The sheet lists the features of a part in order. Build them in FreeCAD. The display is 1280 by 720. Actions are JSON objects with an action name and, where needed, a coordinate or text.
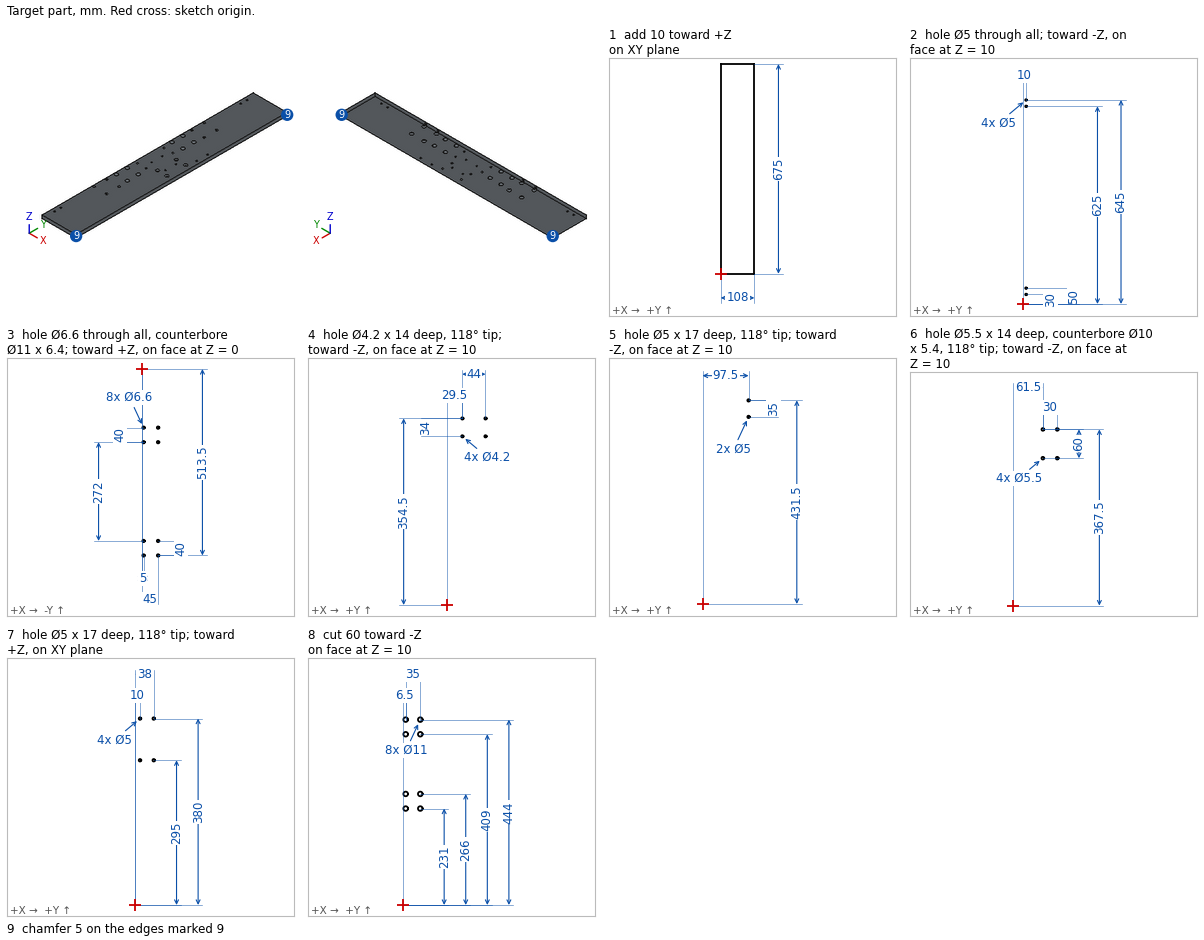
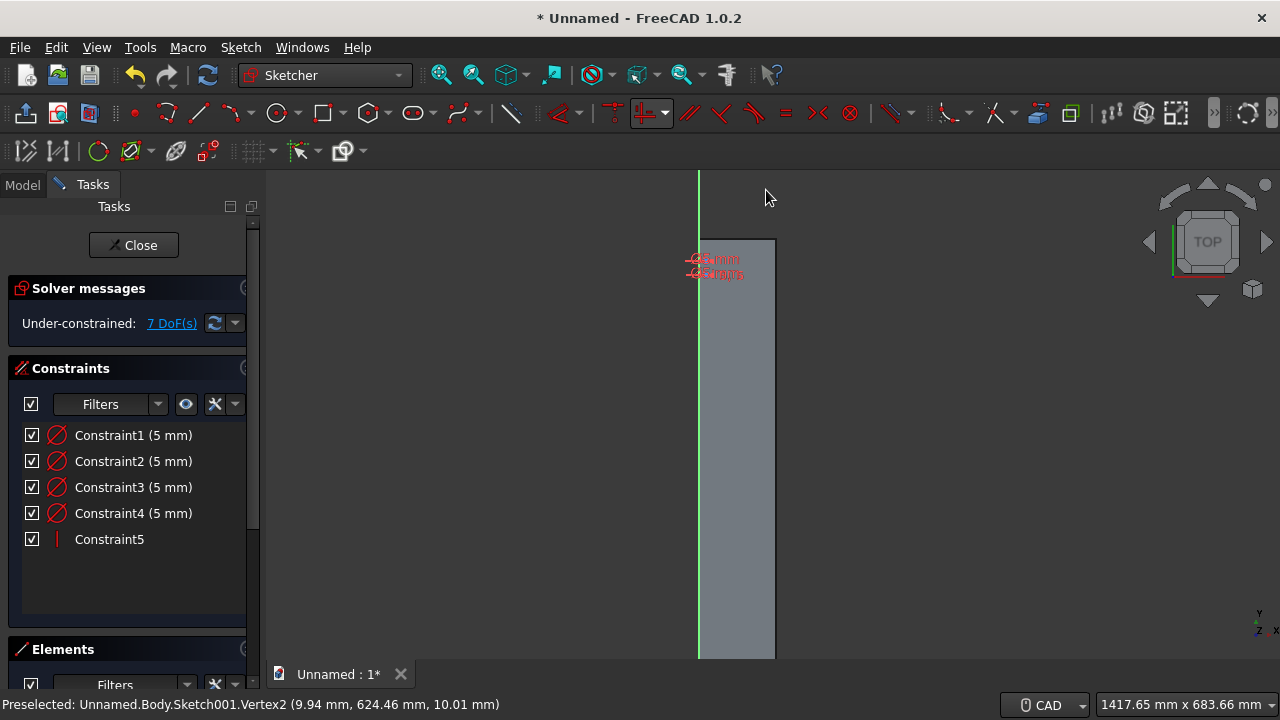
{"action": "left_click", "coordinate": [706, 275]}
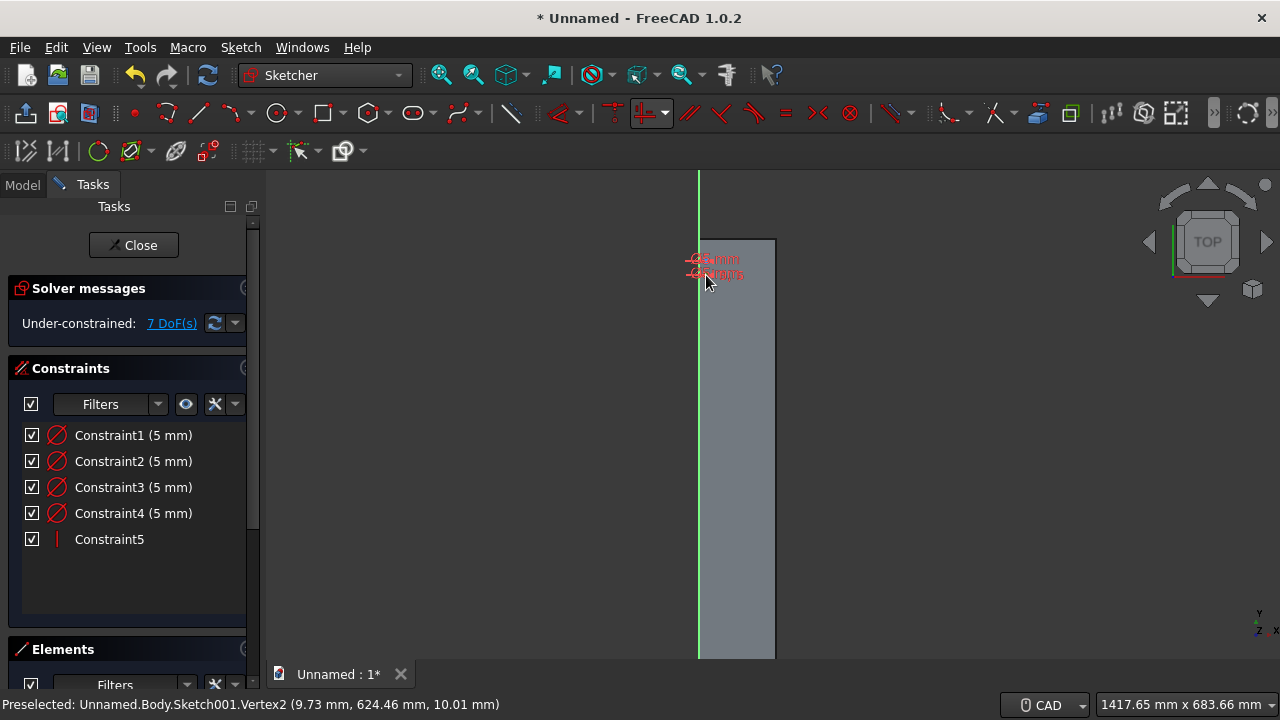
{"action": "scroll", "coordinate": [706, 260], "scroll_direction": "down", "scroll_amount": 2}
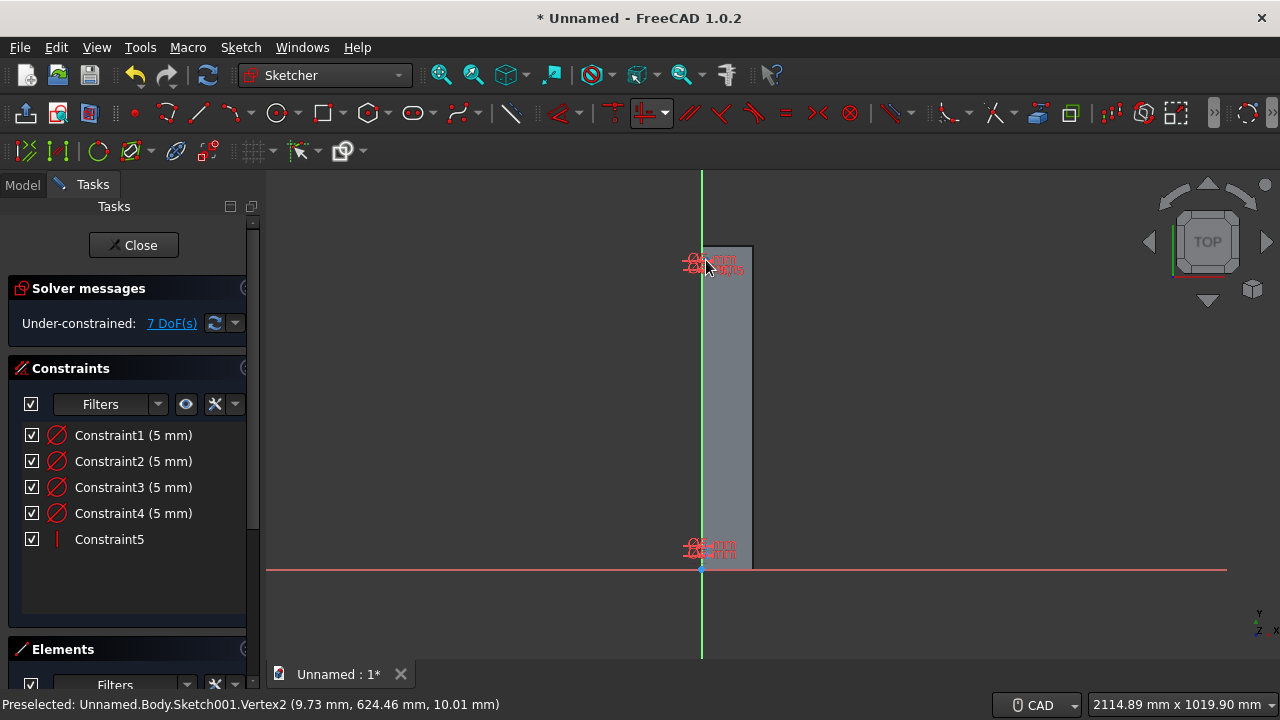
{"action": "scroll", "coordinate": [706, 546], "scroll_direction": "up", "scroll_amount": 2}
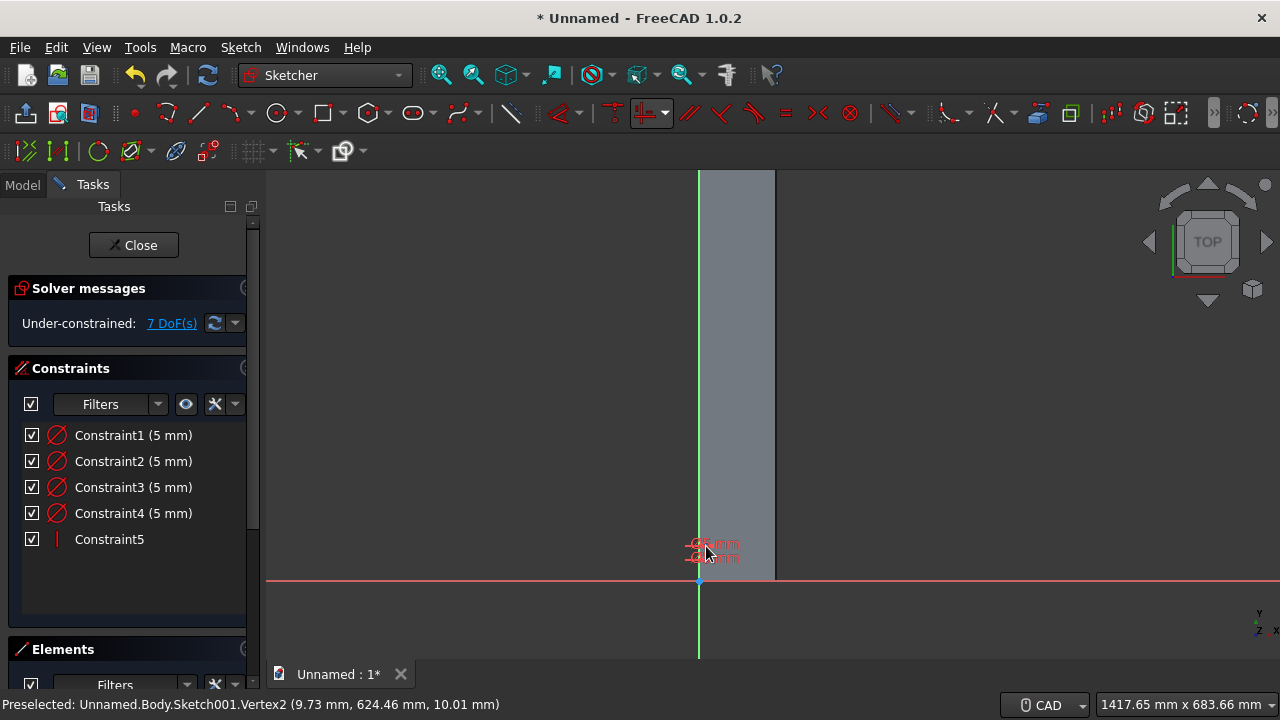
{"action": "left_click", "coordinate": [706, 546]}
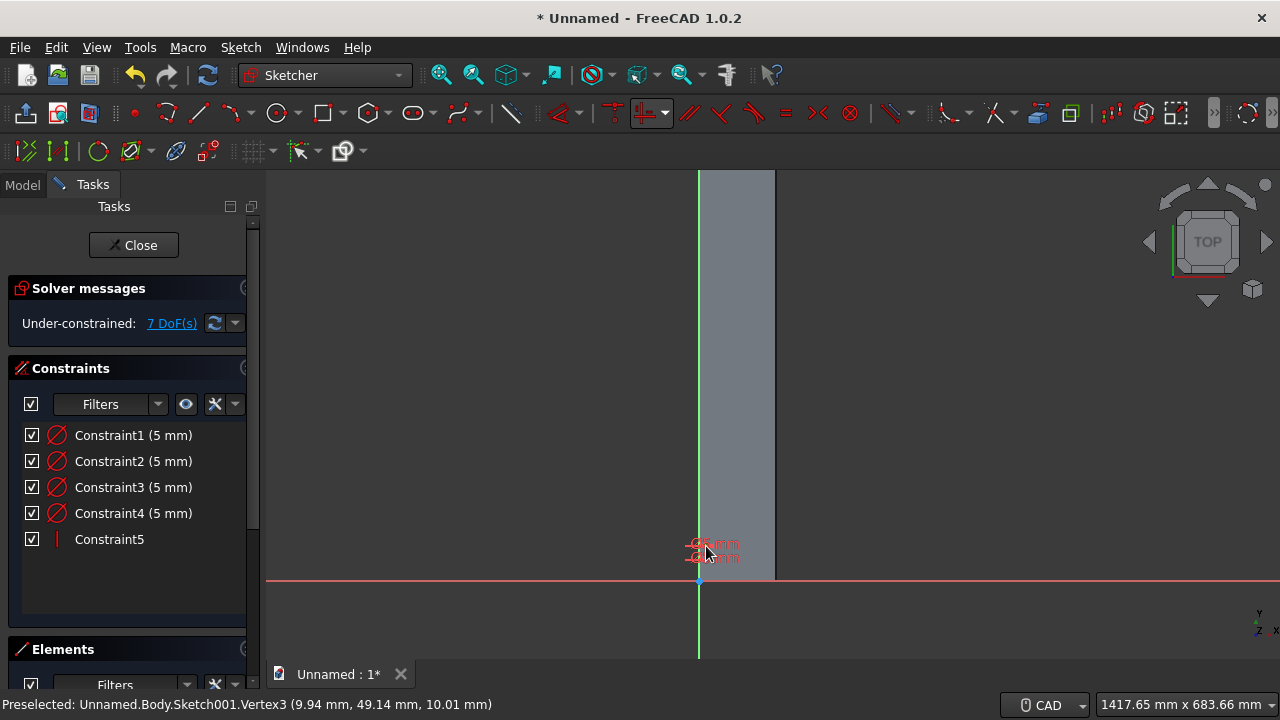
{"action": "key", "text": "v"}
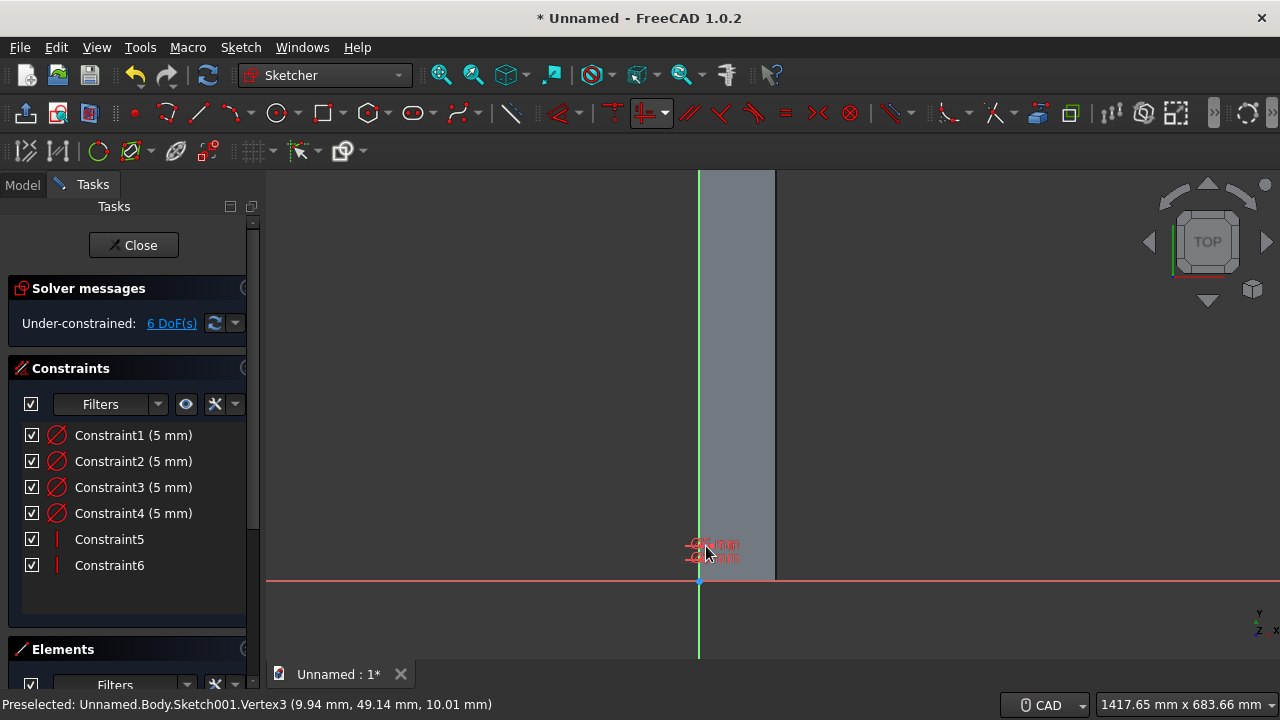
{"action": "left_click", "coordinate": [706, 546]}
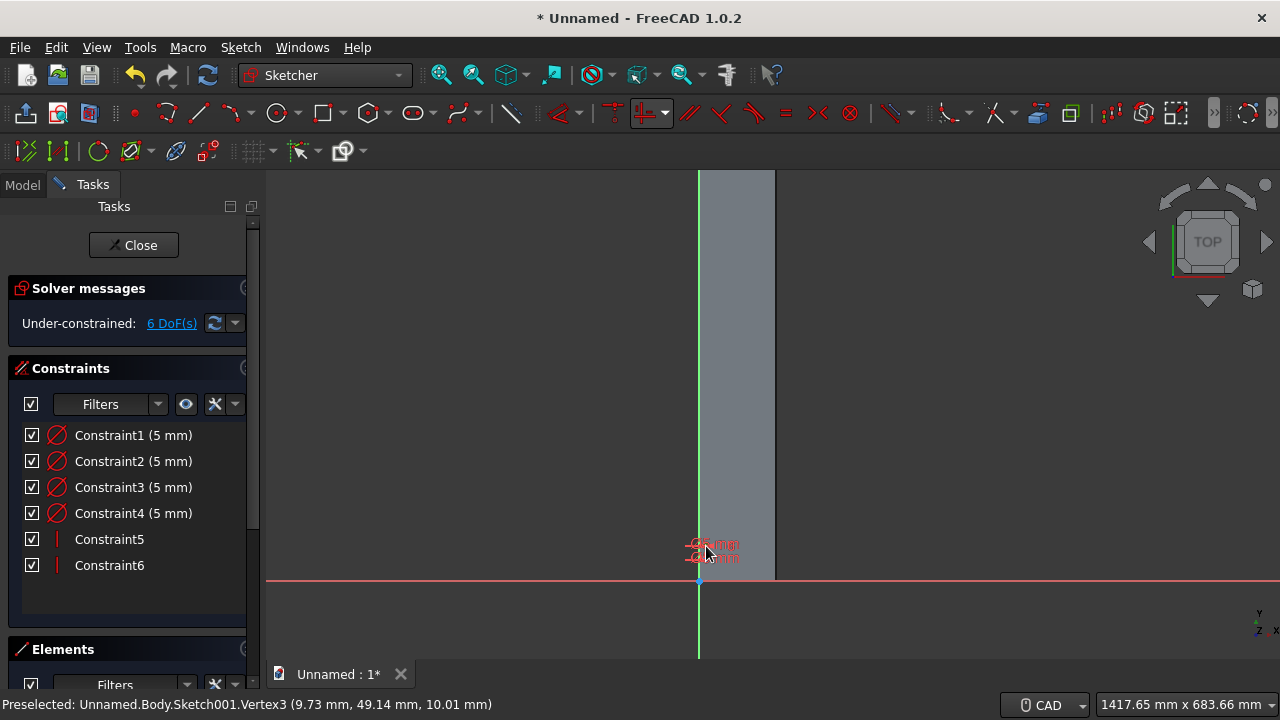
{"action": "left_click", "coordinate": [706, 560]}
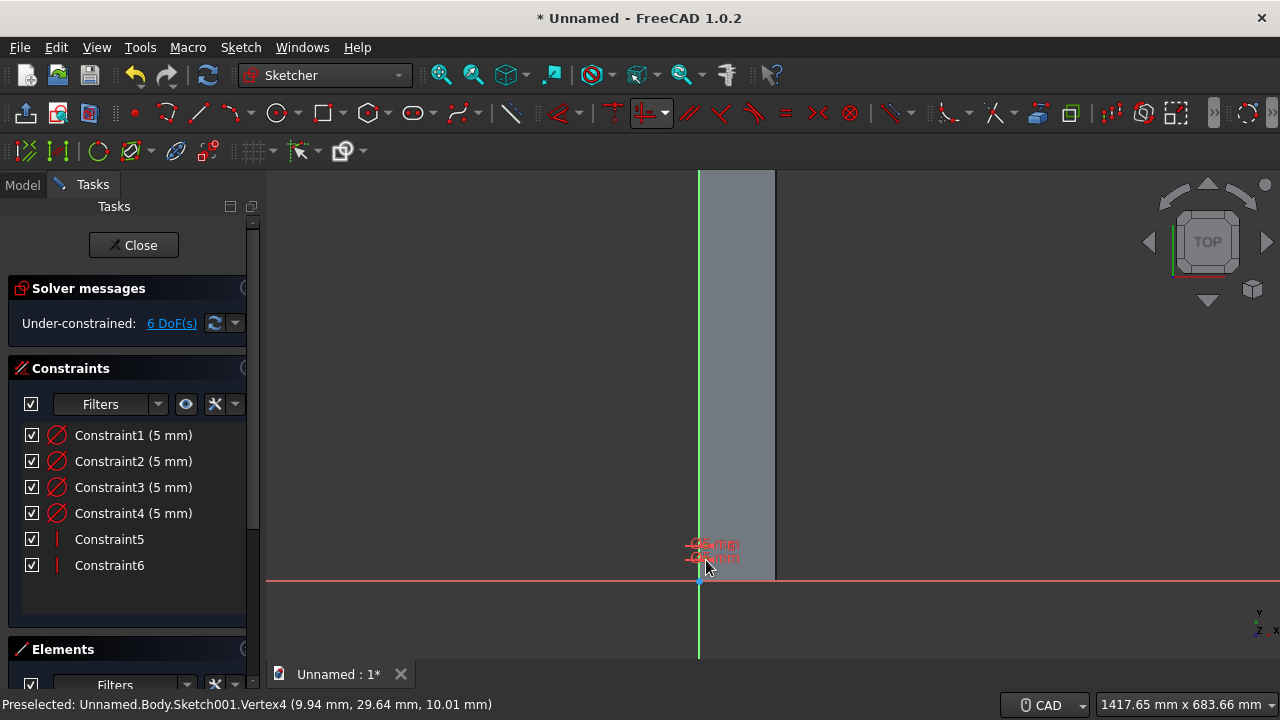
{"action": "key", "text": "v"}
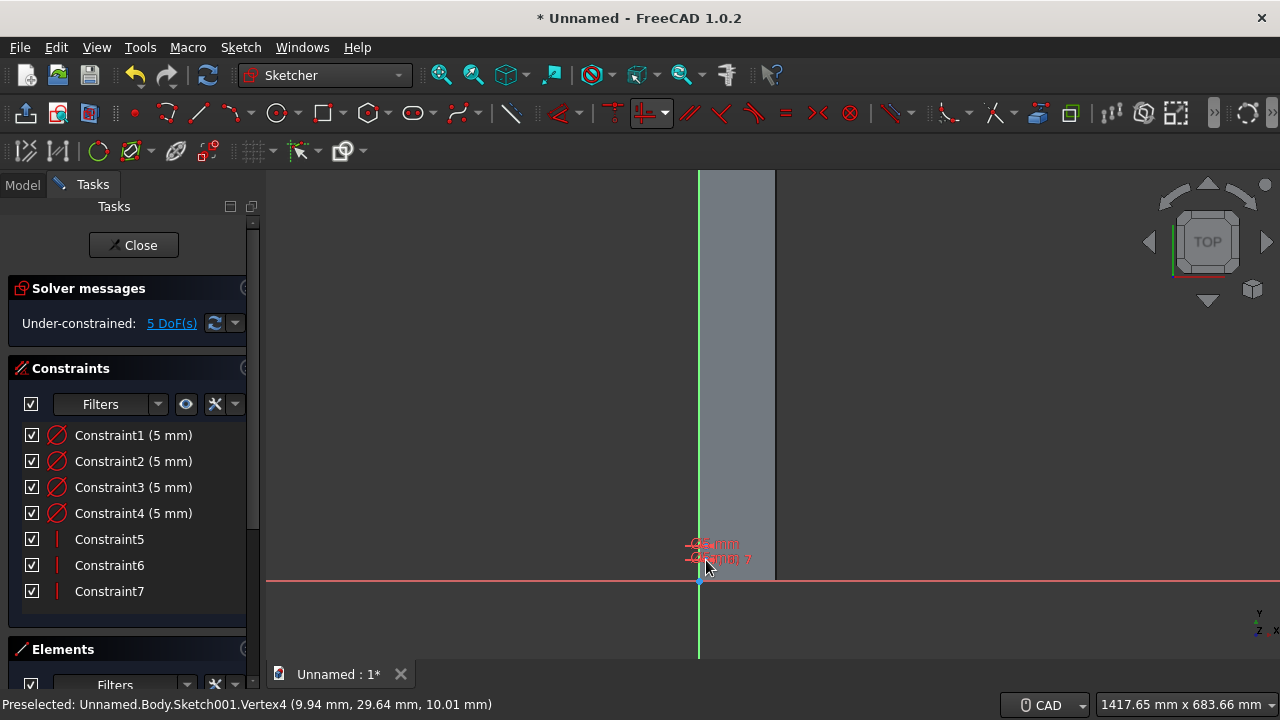
{"action": "left_click", "coordinate": [558, 114]}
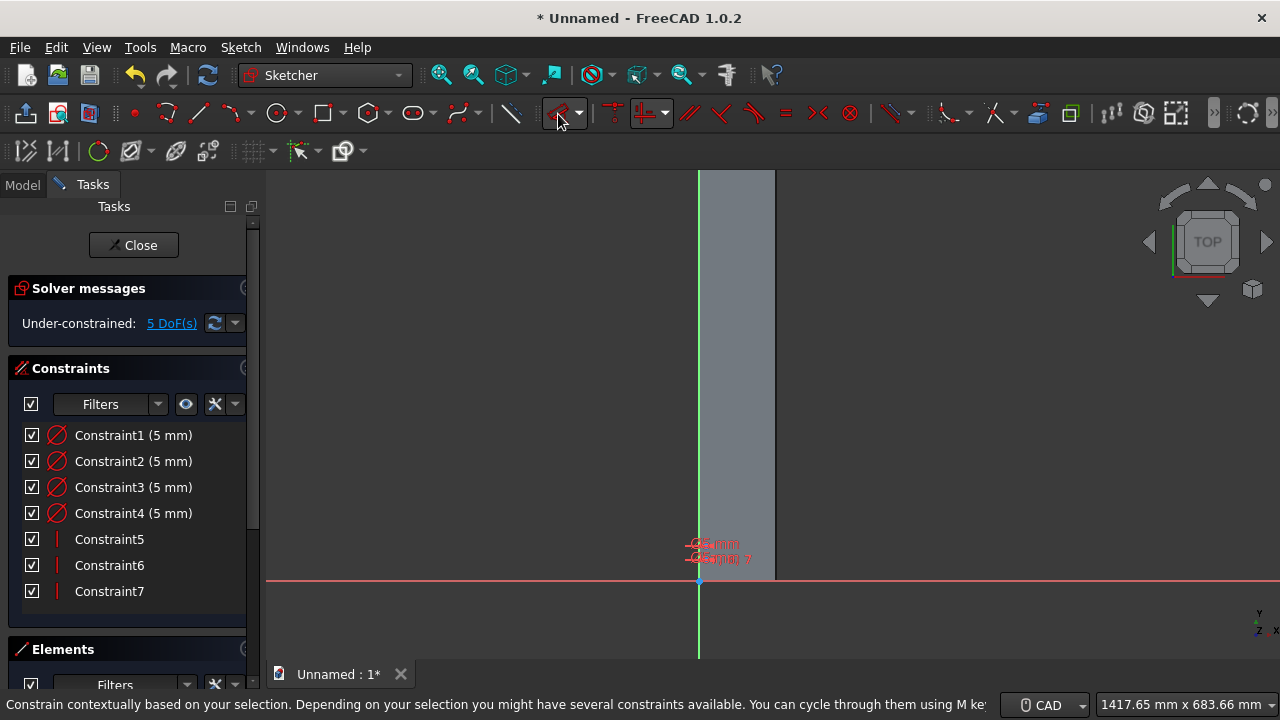
{"action": "scroll", "coordinate": [706, 546], "scroll_direction": "down", "scroll_amount": 2}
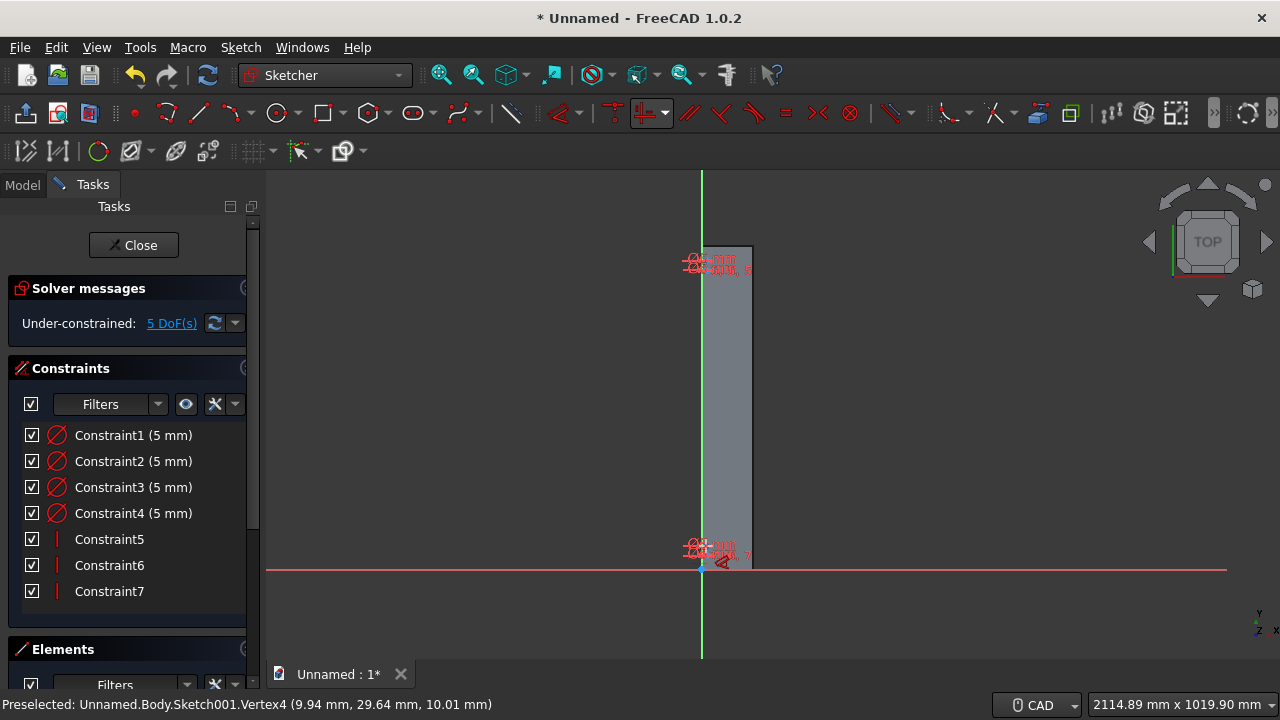
{"action": "scroll", "coordinate": [706, 261], "scroll_direction": "up", "scroll_amount": 11}